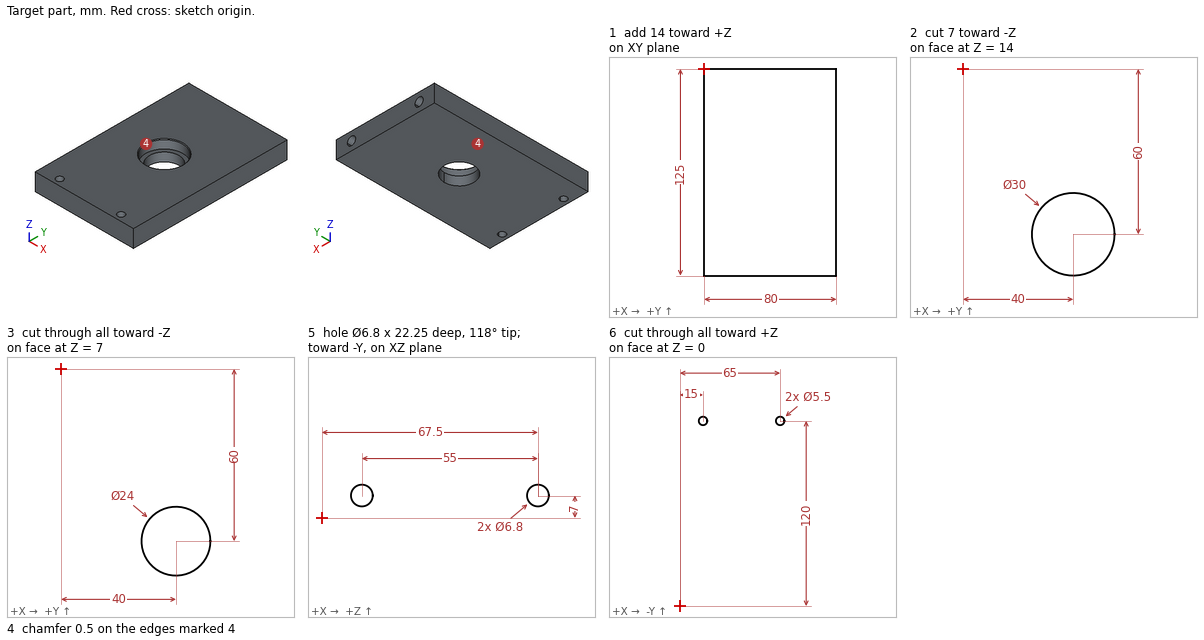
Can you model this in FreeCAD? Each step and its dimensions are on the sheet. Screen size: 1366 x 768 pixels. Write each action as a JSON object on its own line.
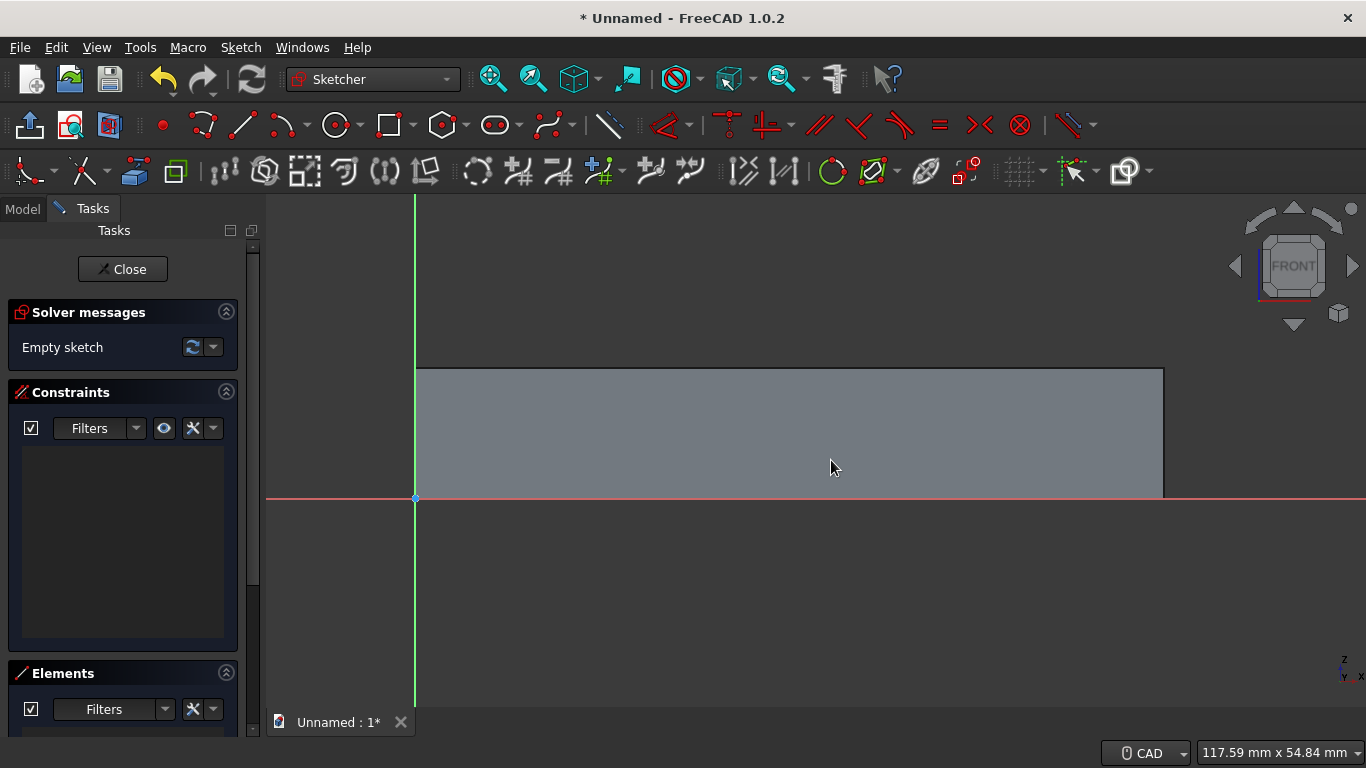
{"action": "key", "text": "g c"}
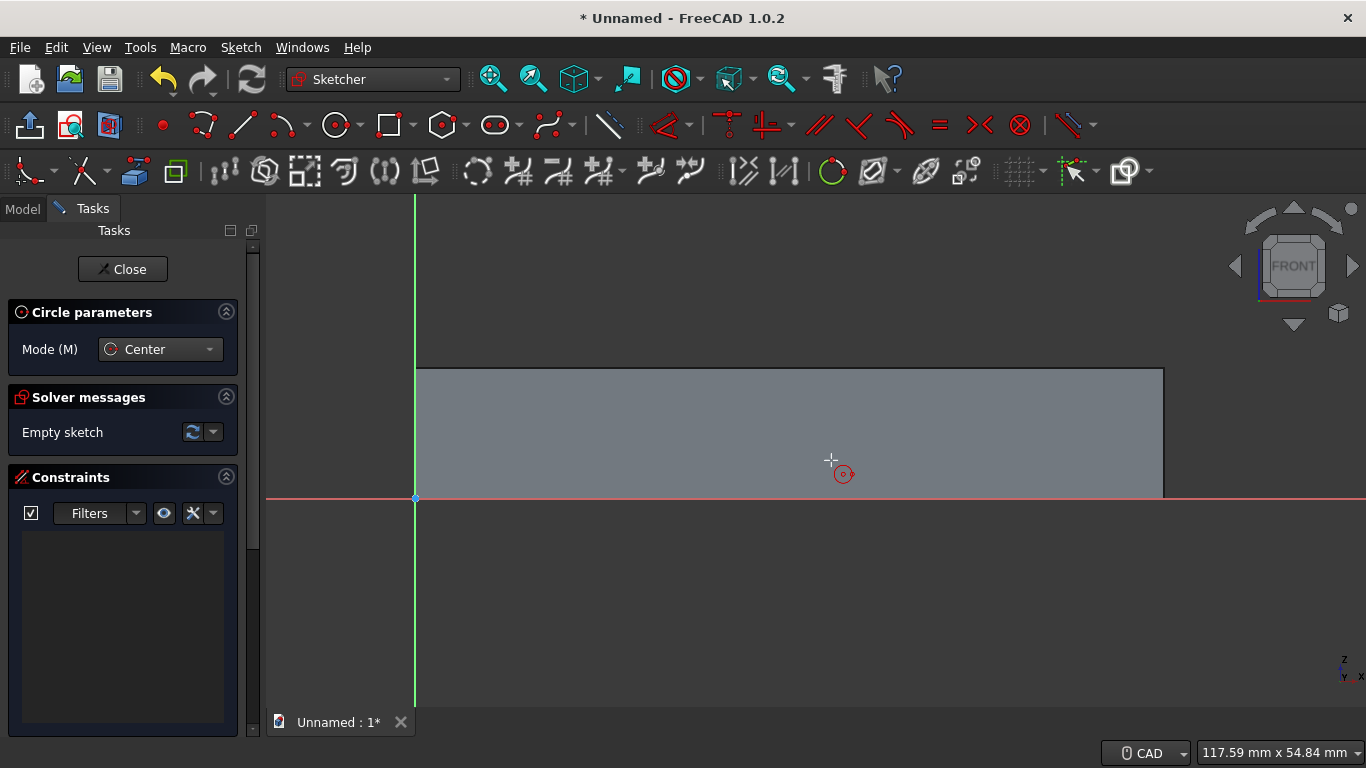
{"action": "left_click", "coordinate": [1047, 433]}
{"action": "left_click", "coordinate": [1069, 411]}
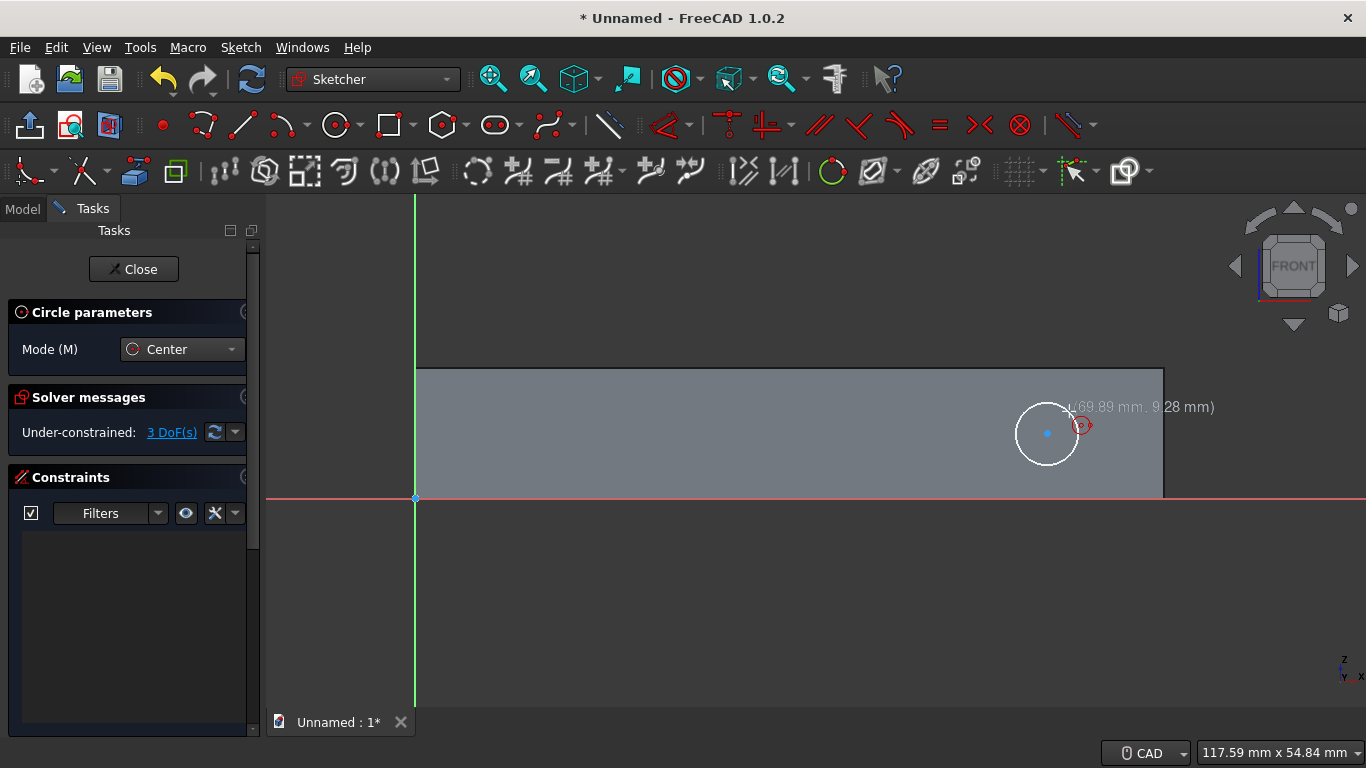
{"action": "left_click", "coordinate": [532, 433]}
{"action": "left_click", "coordinate": [555, 411]}
{"action": "key", "text": "Escape"}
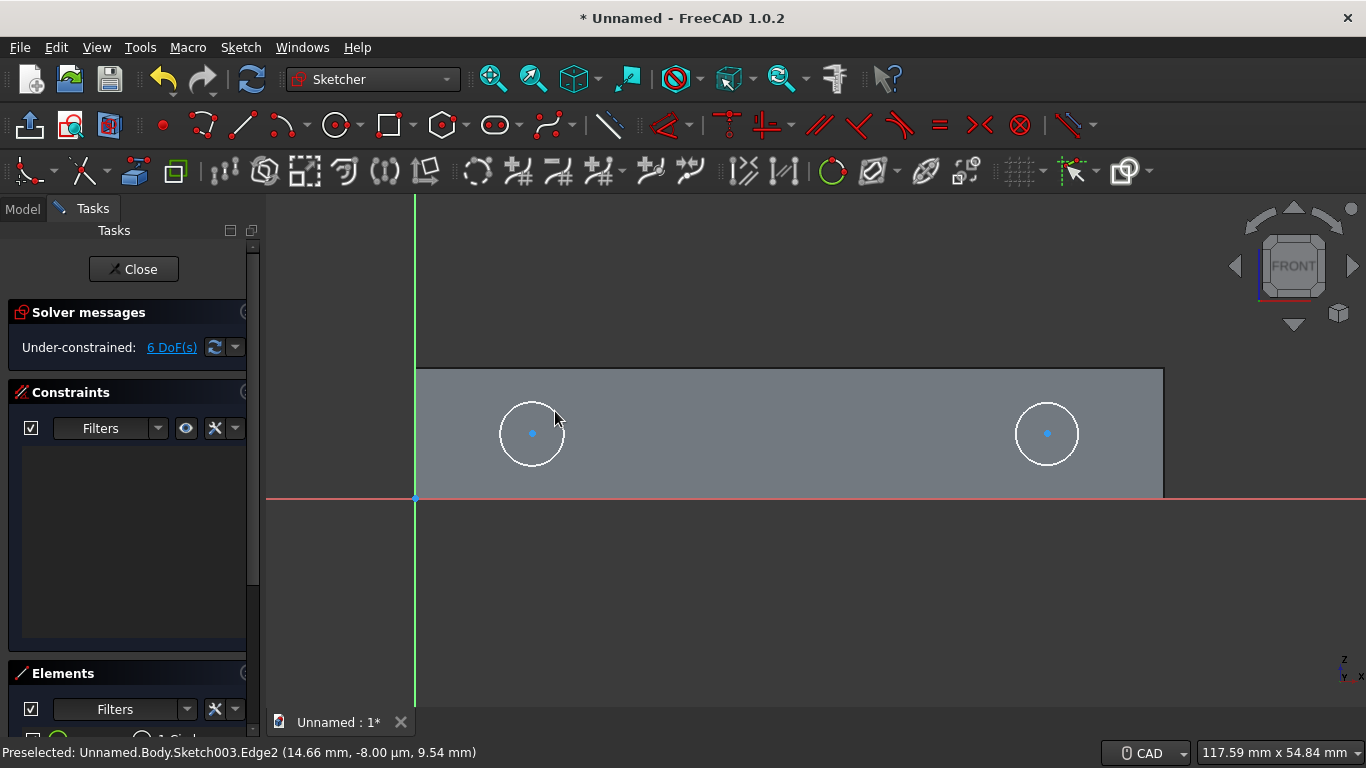
{"action": "left_click", "coordinate": [1069, 412]}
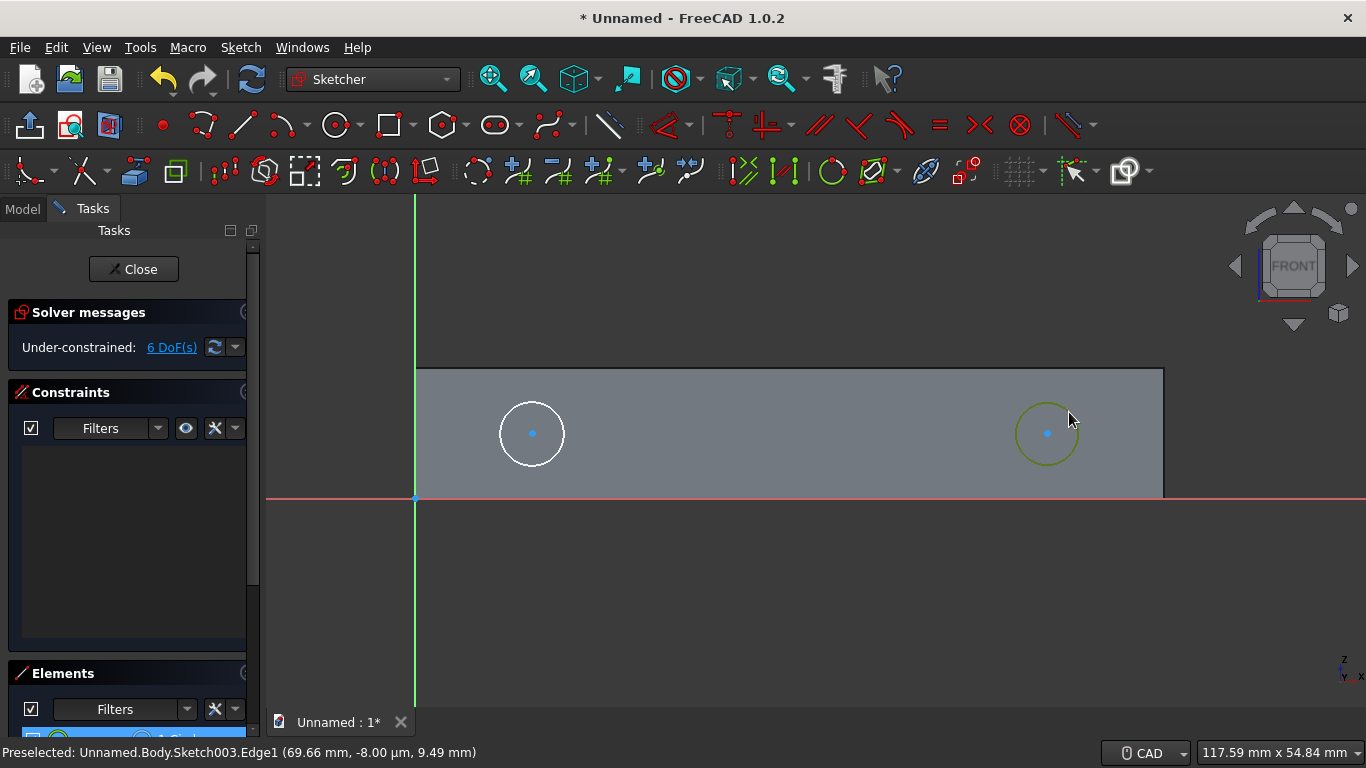
{"action": "left_click", "coordinate": [554, 411]}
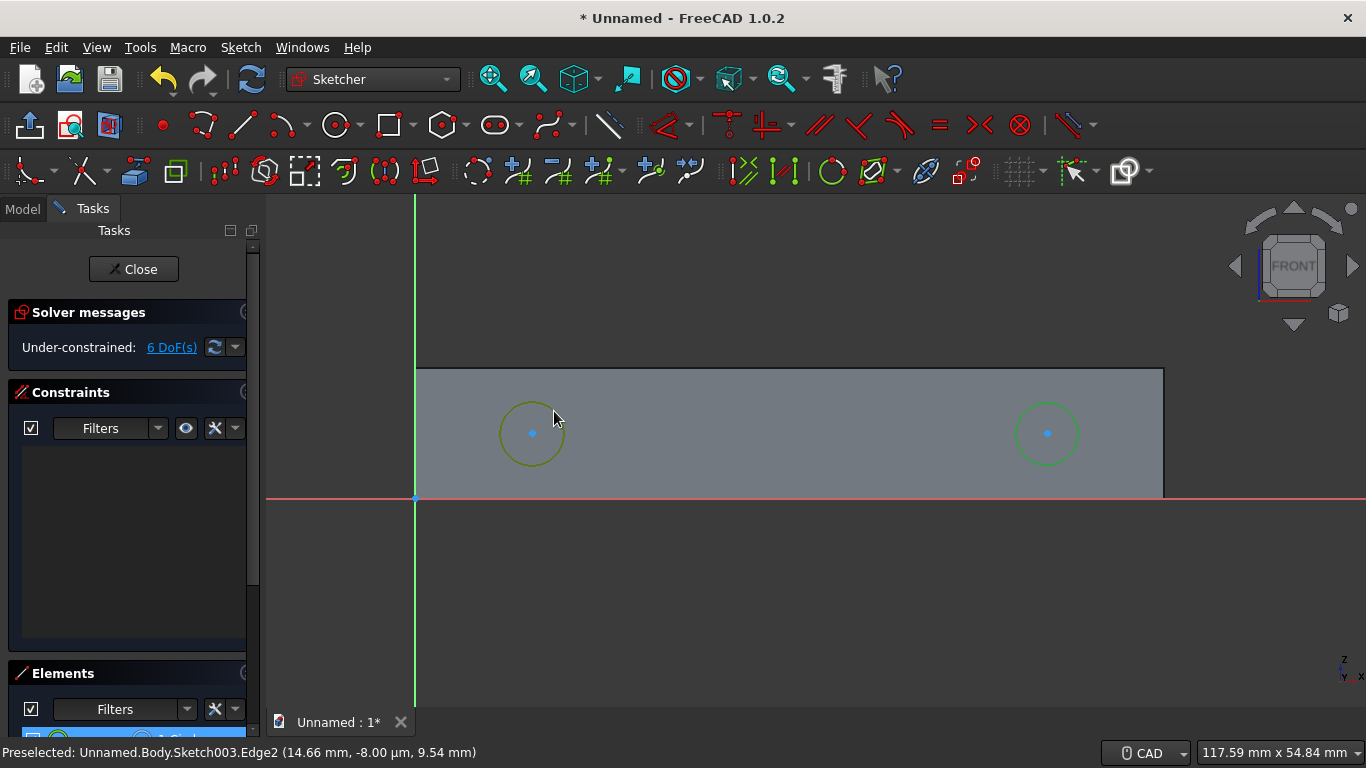
{"action": "left_click", "coordinate": [940, 126]}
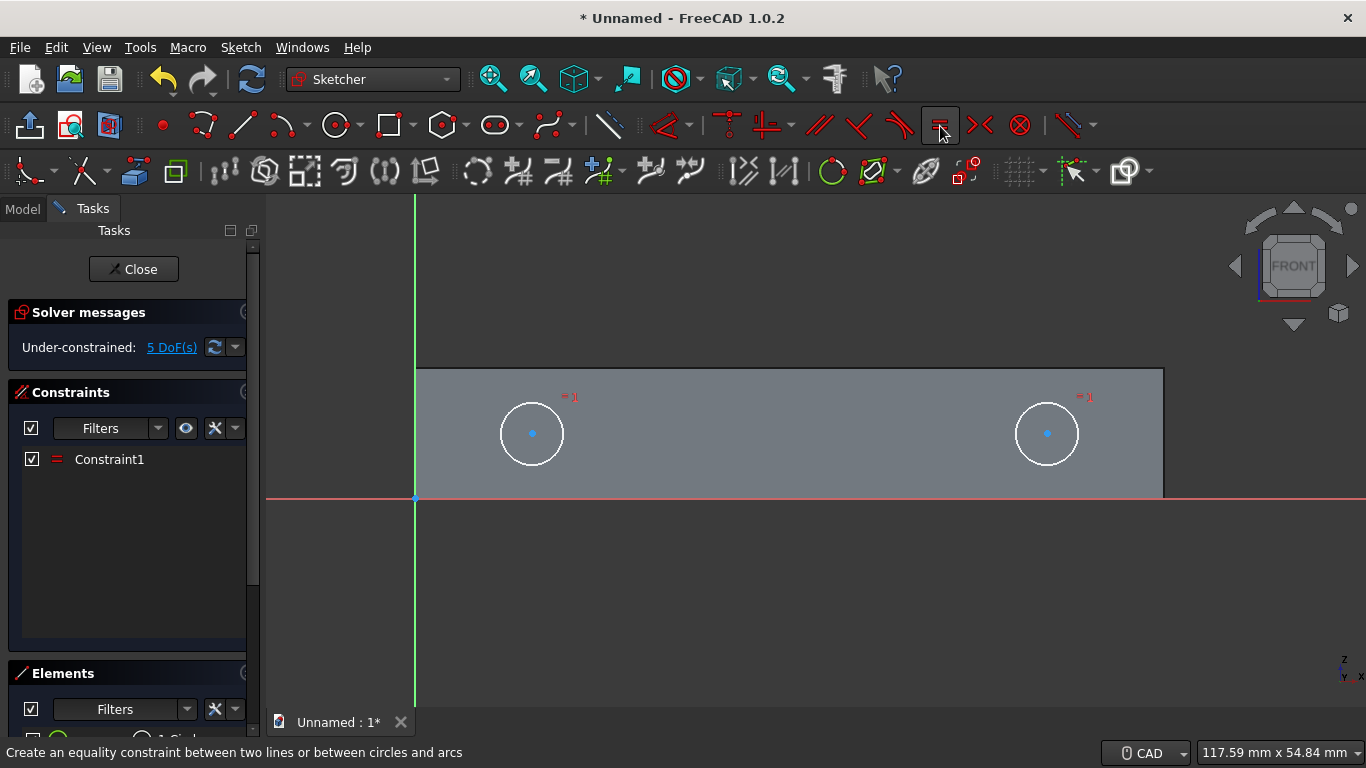
{"action": "left_click", "coordinate": [1047, 434]}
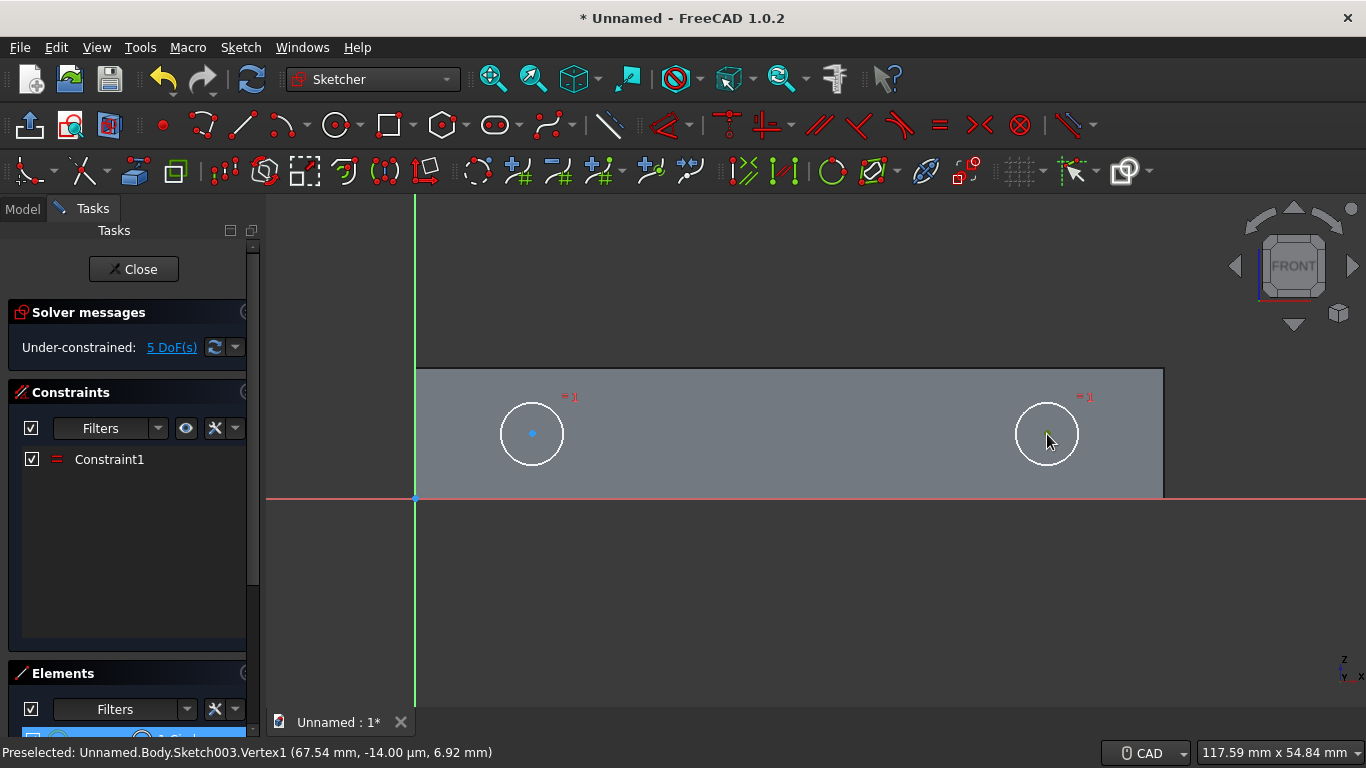
{"action": "left_click", "coordinate": [532, 434]}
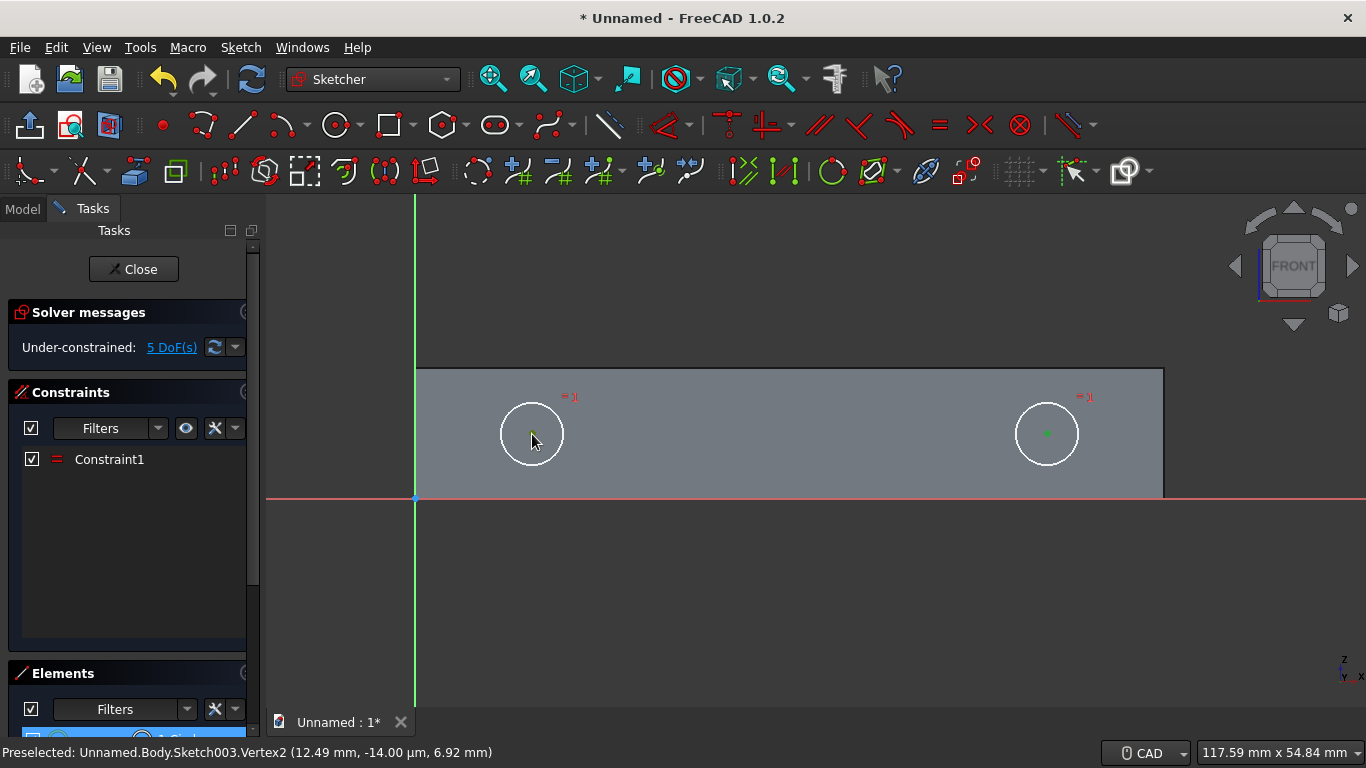
{"action": "left_click", "coordinate": [794, 126]}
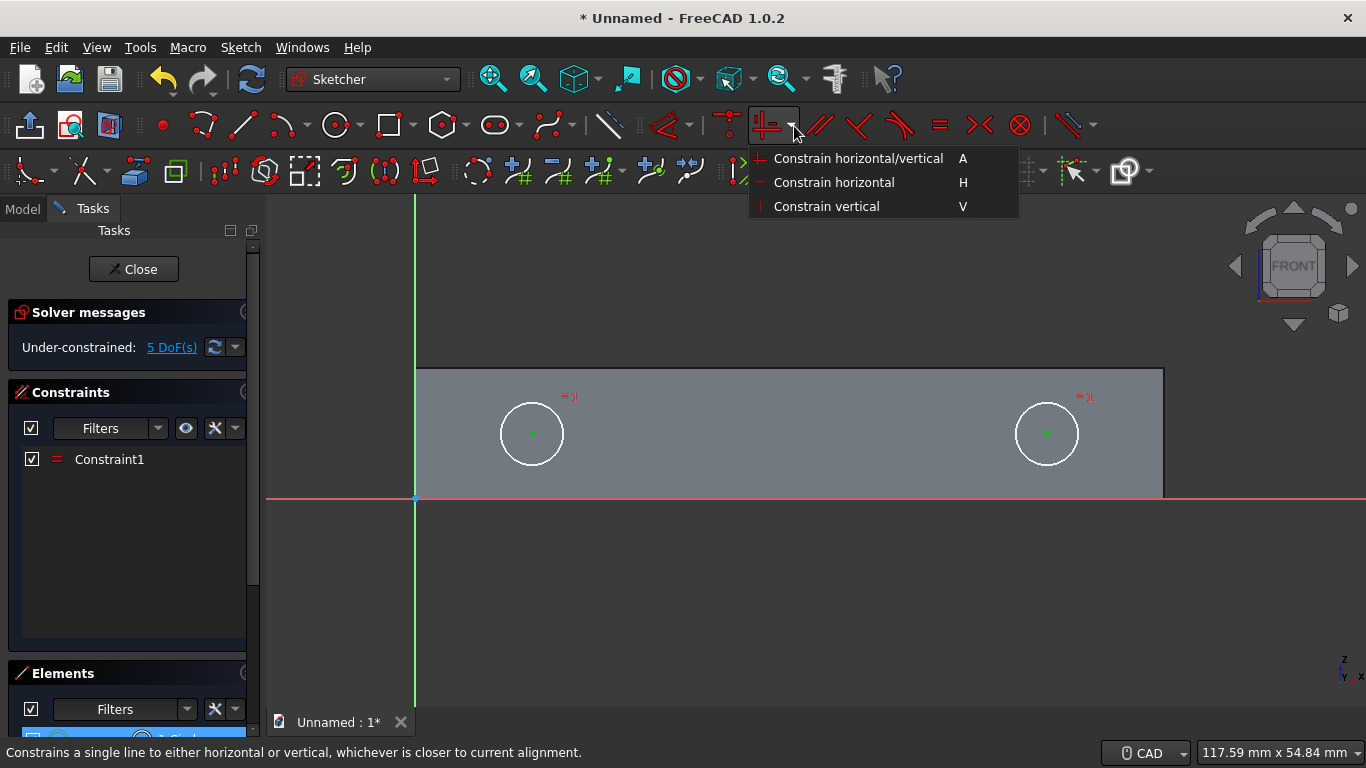
{"action": "left_click", "coordinate": [884, 182]}